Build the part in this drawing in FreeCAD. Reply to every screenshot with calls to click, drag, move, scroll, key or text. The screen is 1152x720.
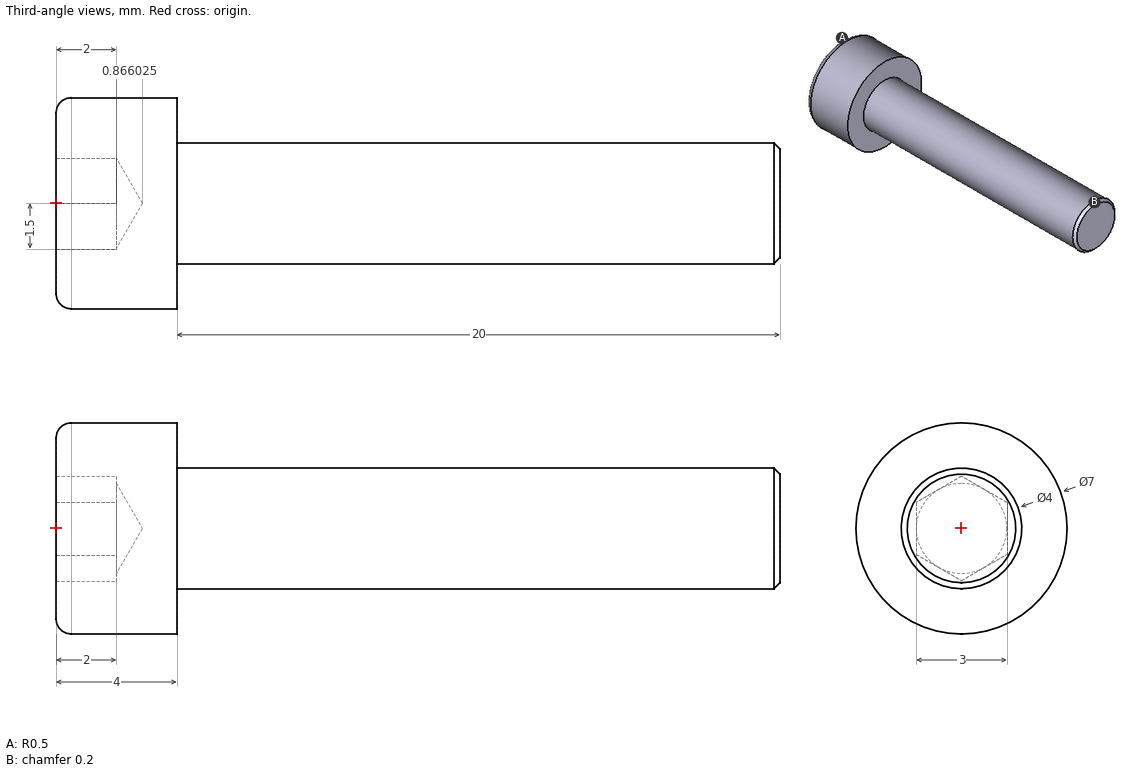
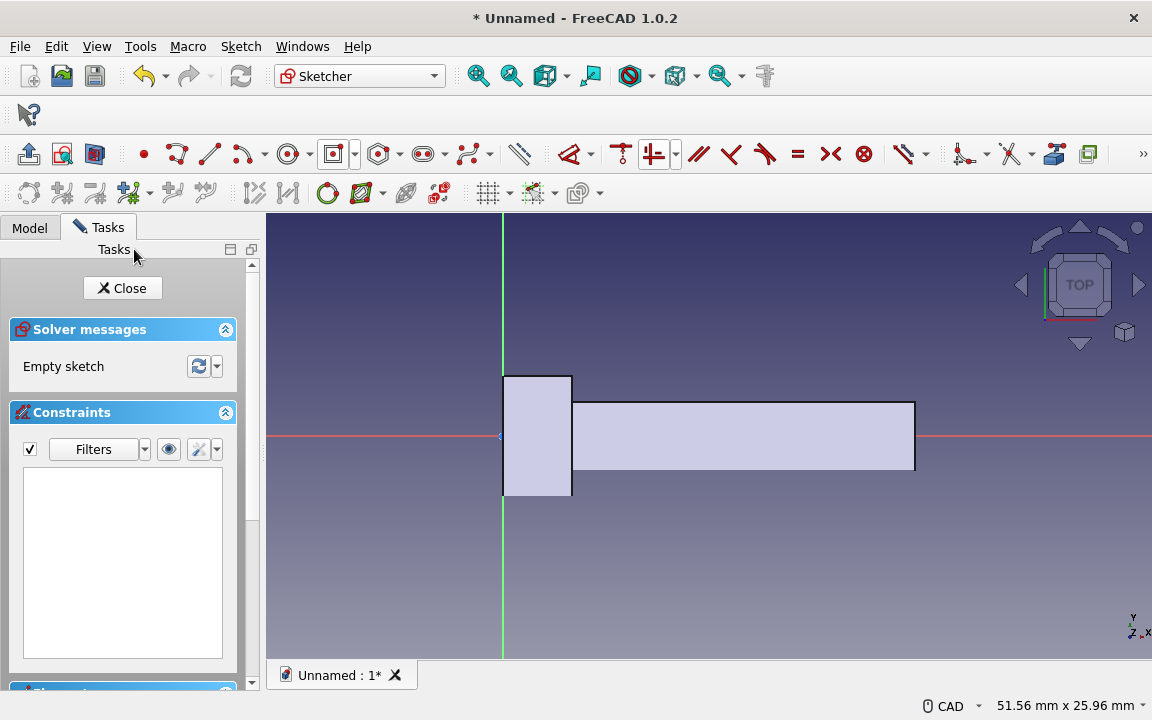
click(95, 154)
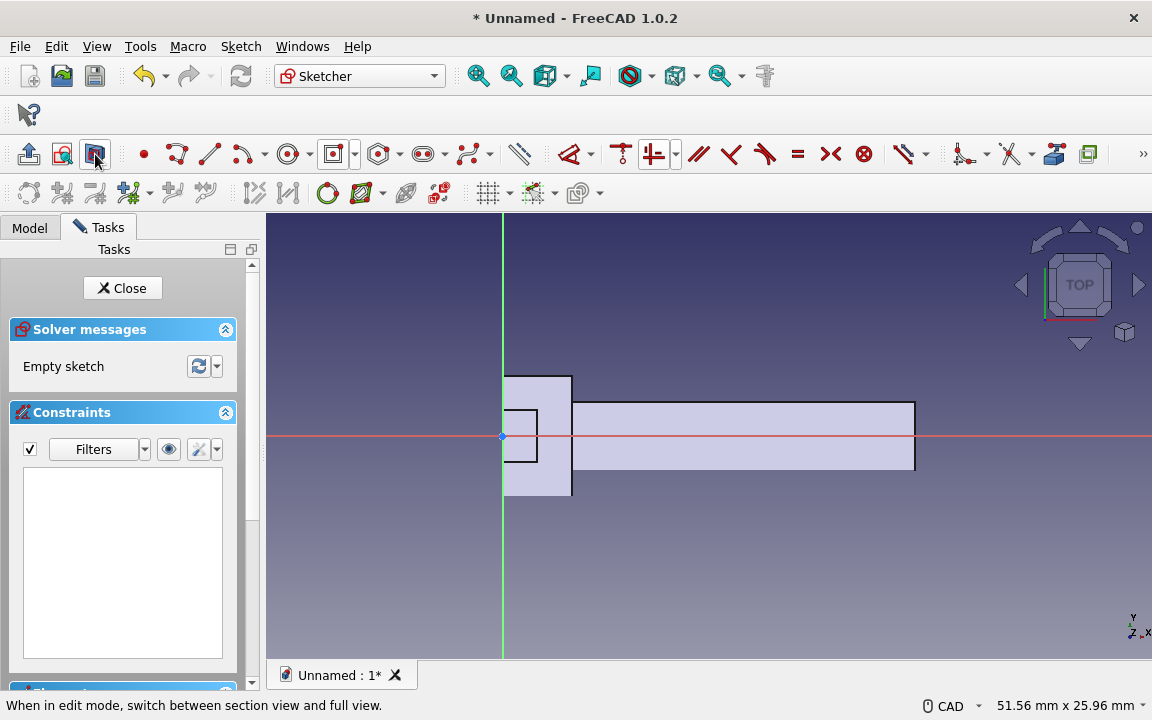
scroll(513, 451, up, 11)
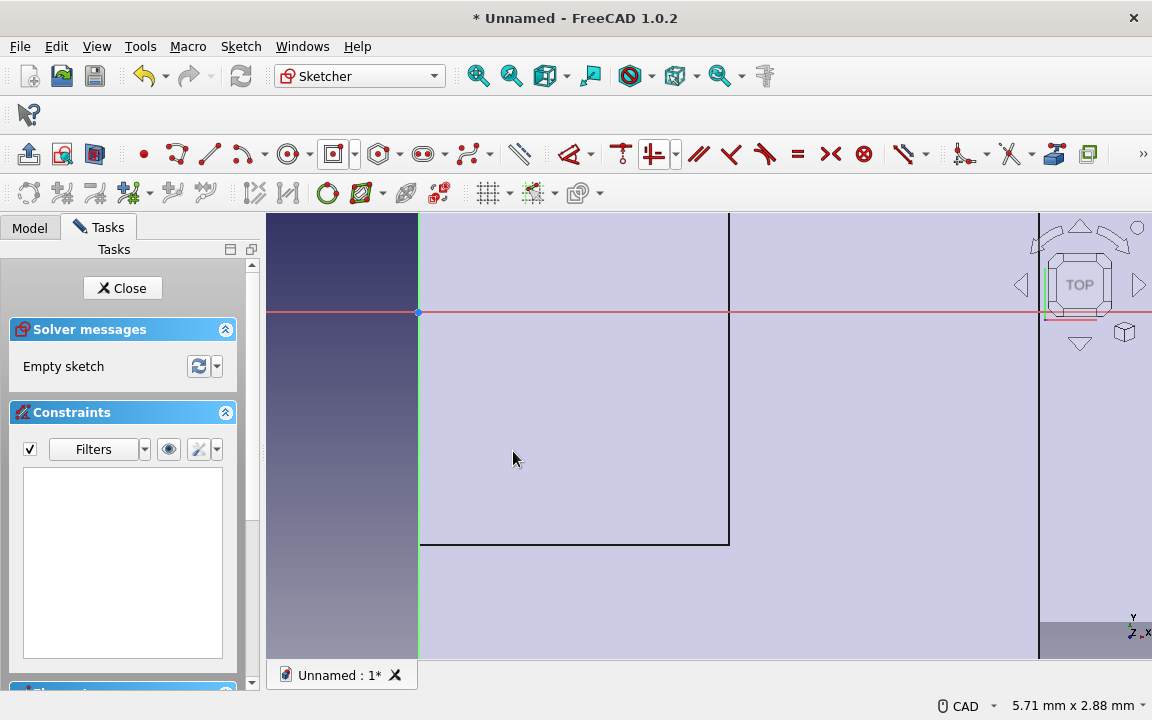
click(177, 154)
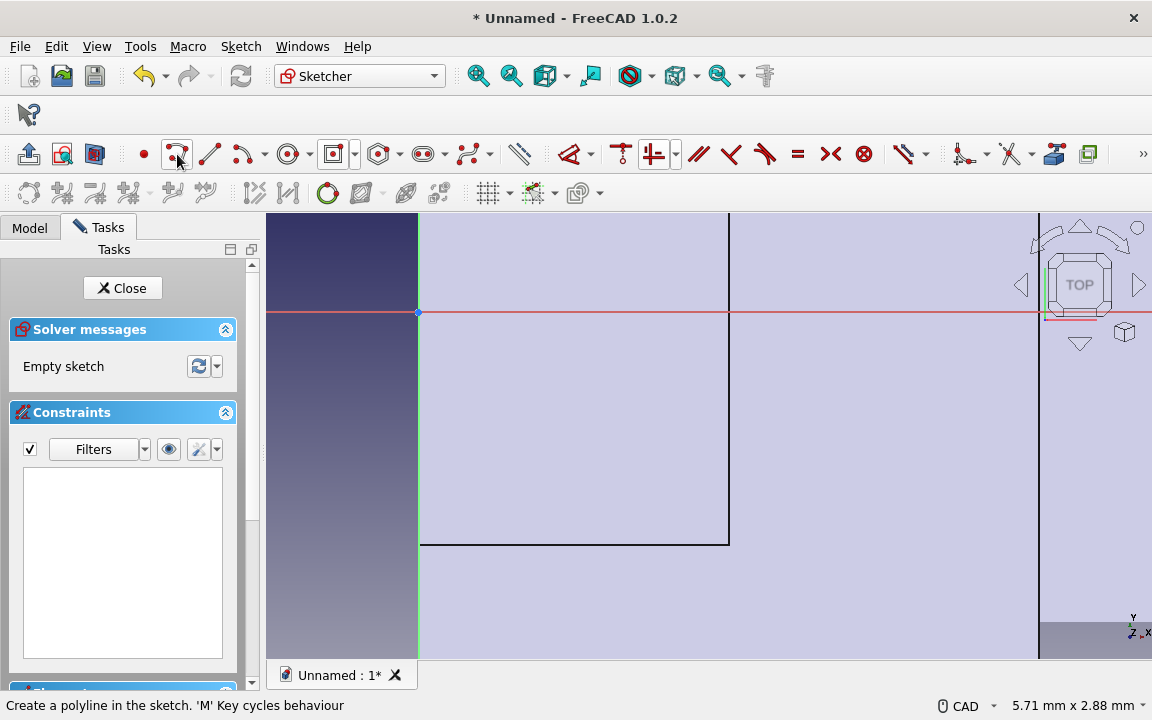
click(729, 312)
click(729, 545)
click(863, 321)
click(729, 312)
key(Escape)
key(Escape)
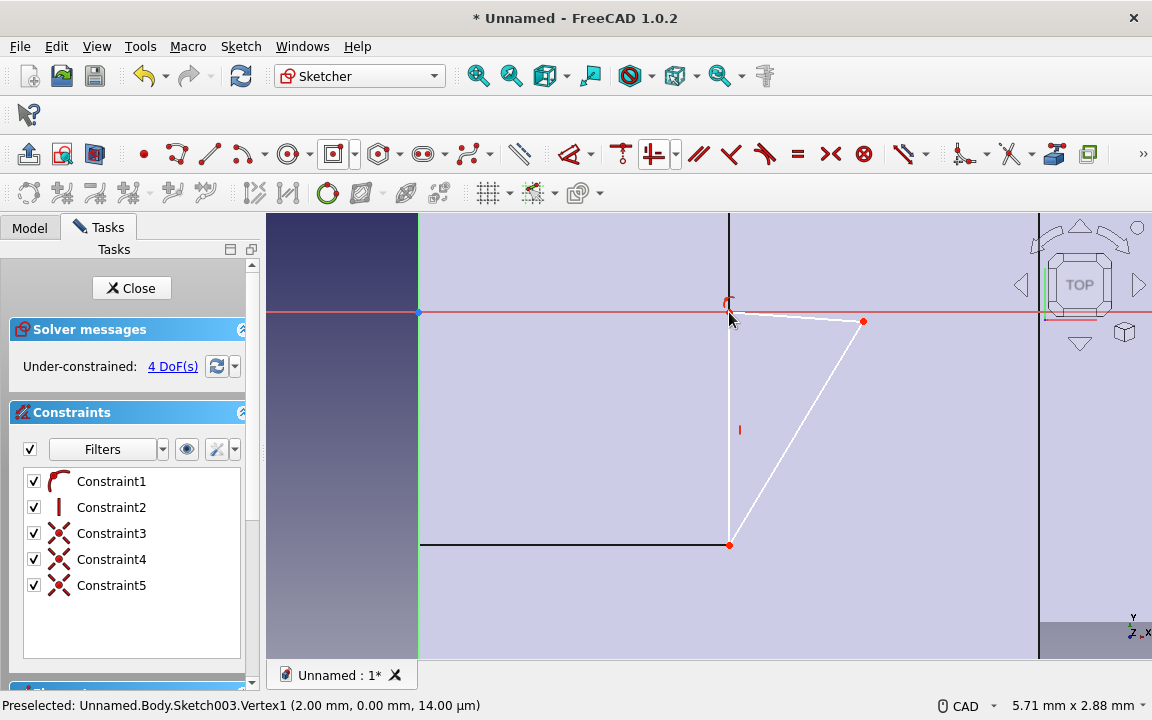
click(769, 315)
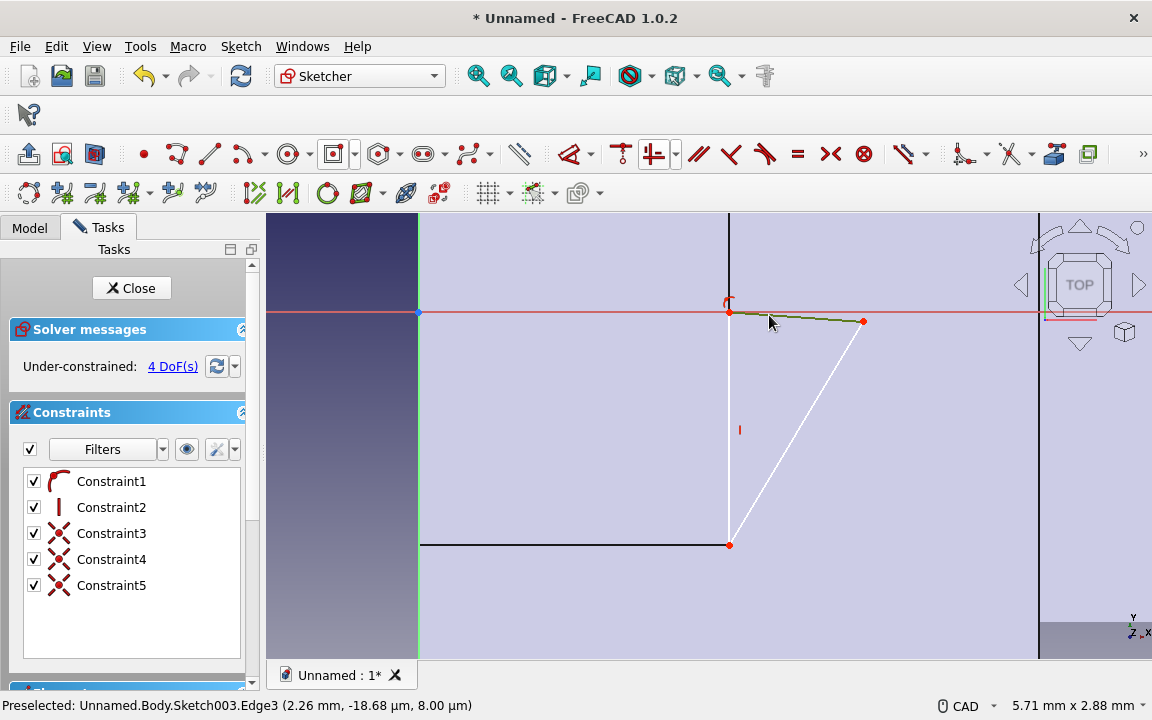
click(676, 154)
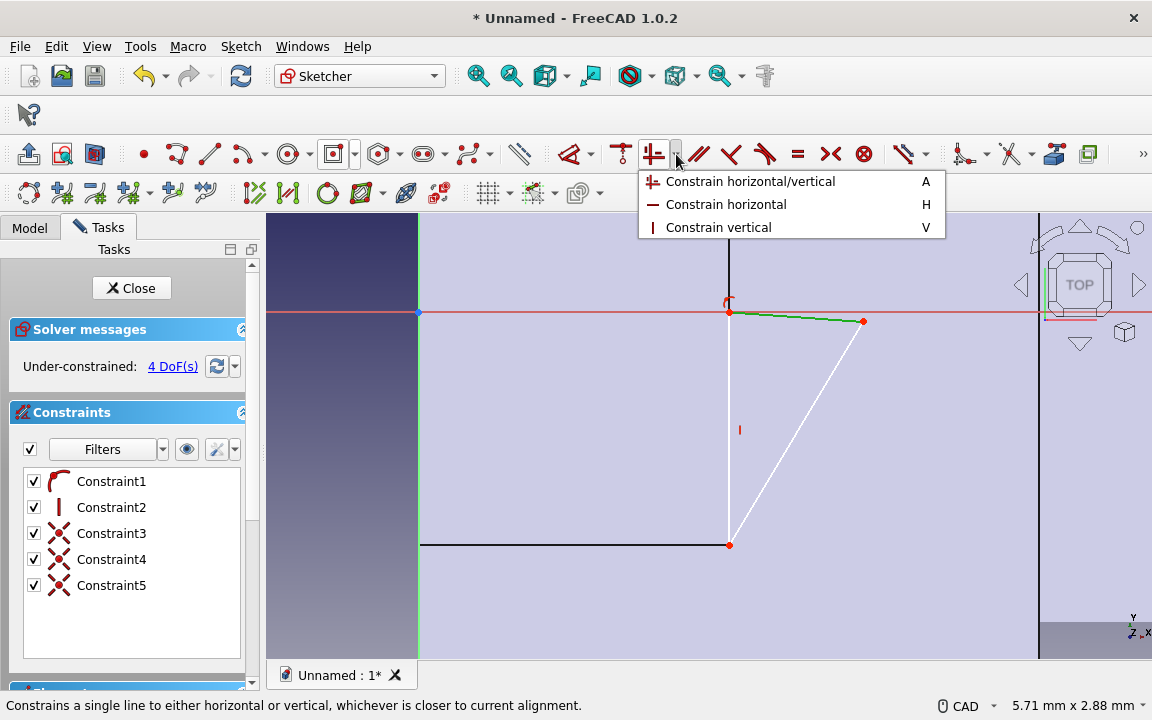
click(792, 204)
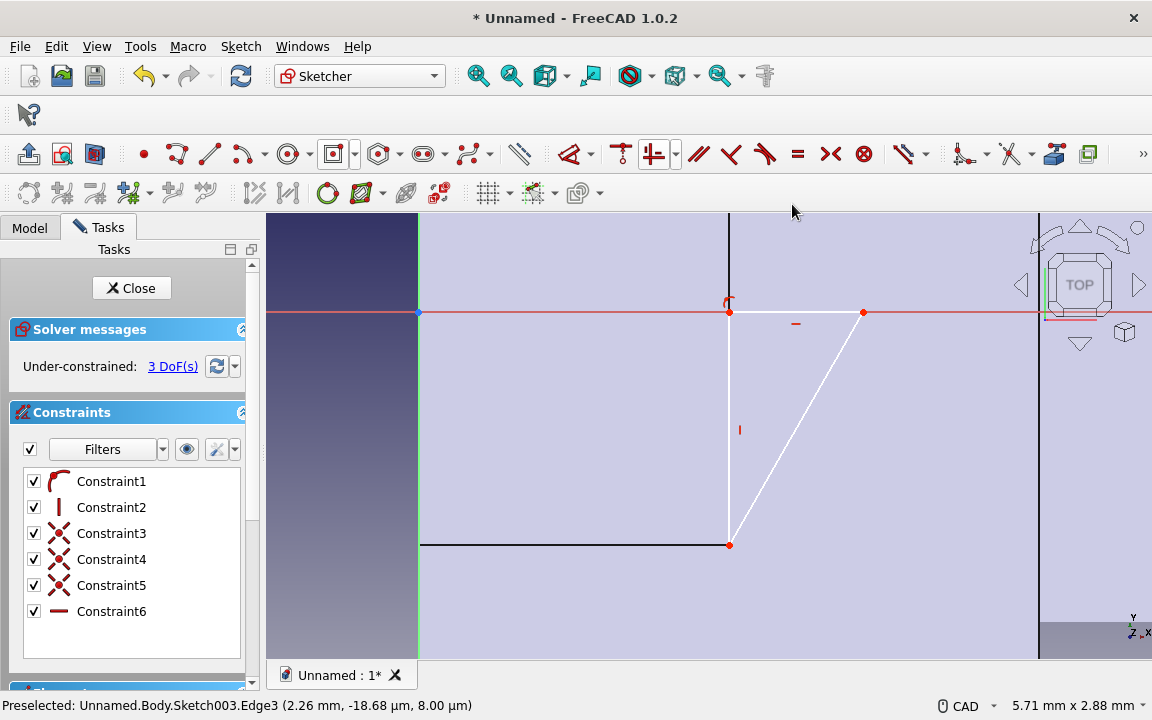
click(568, 154)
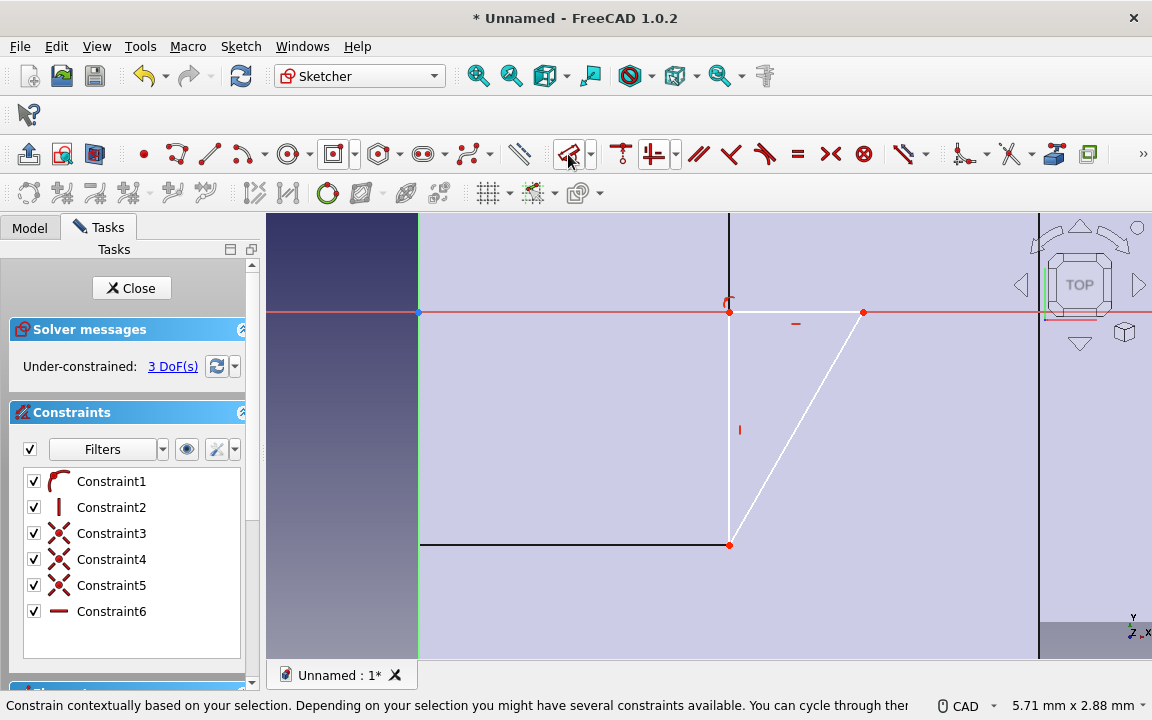
click(729, 312)
click(574, 278)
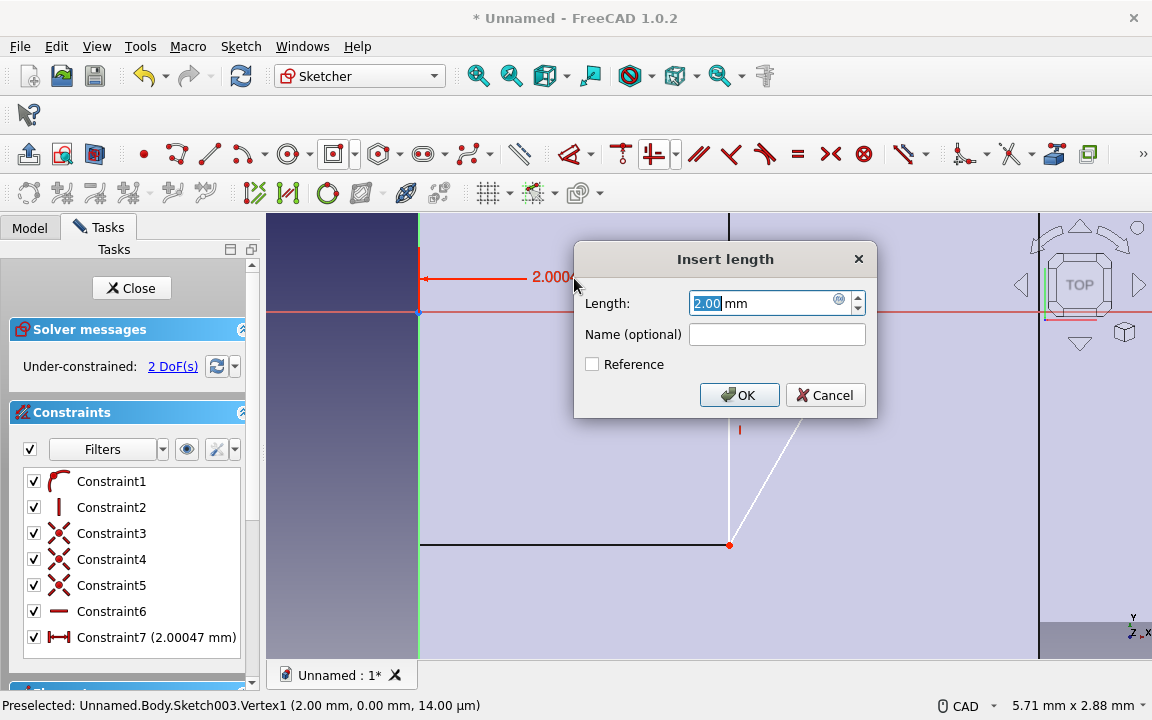
text(2)
key(Return)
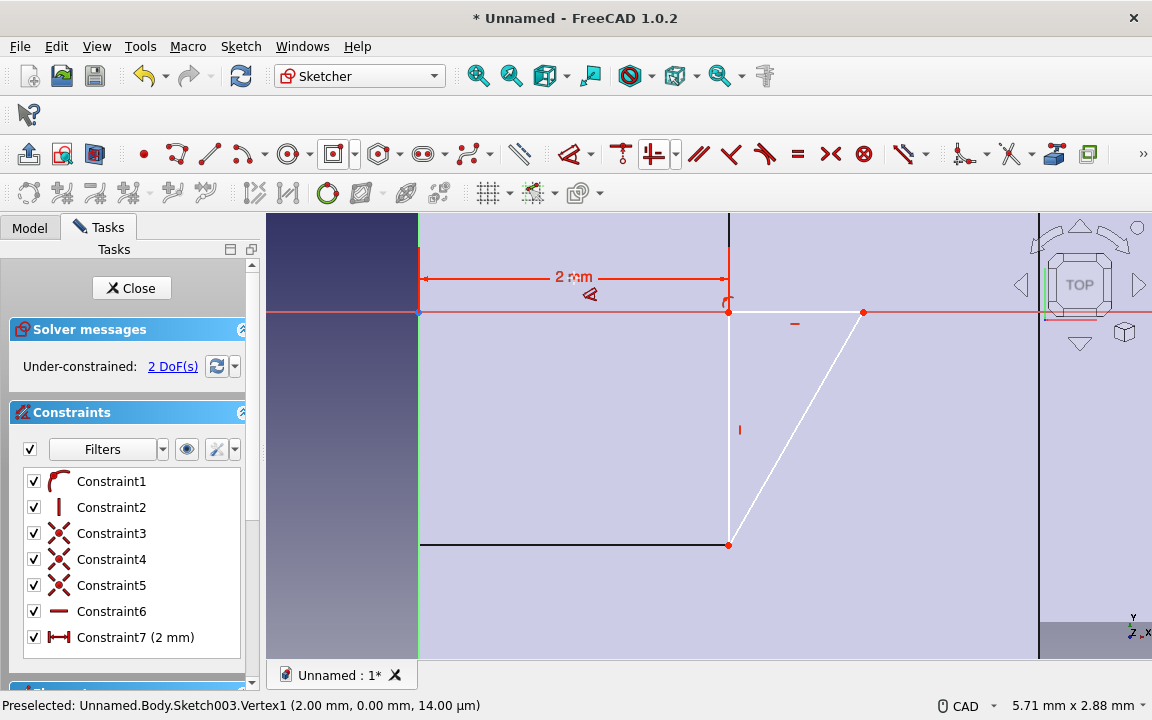
click(729, 382)
click(763, 429)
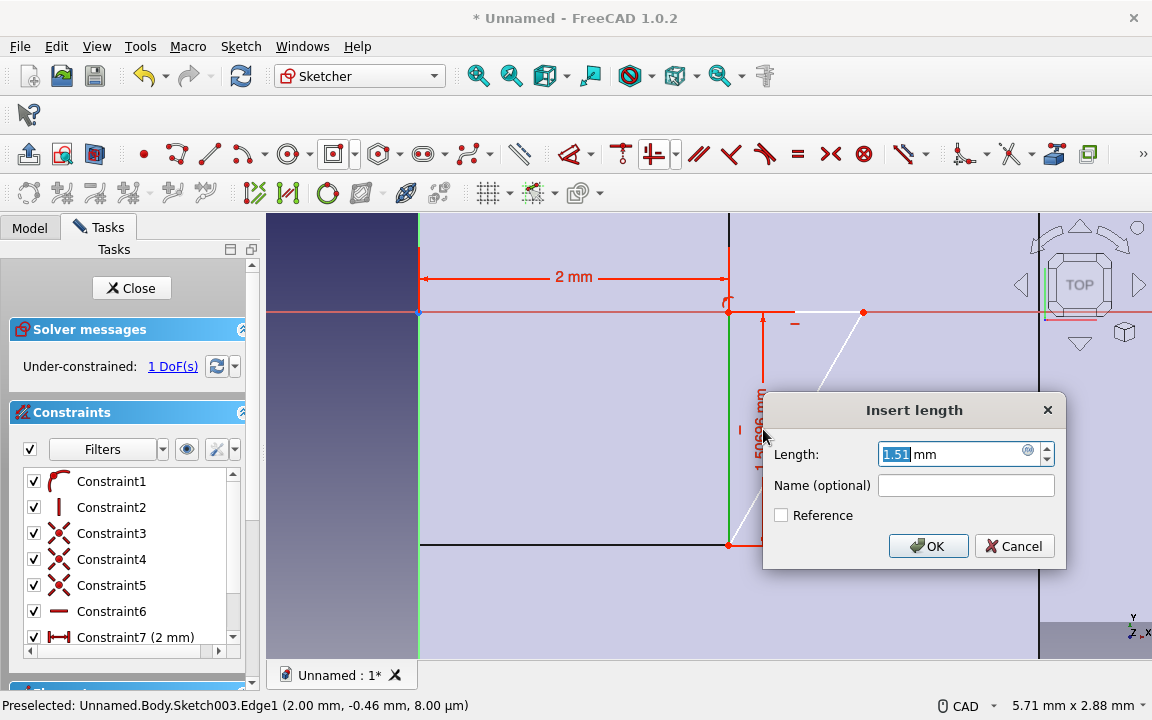
text(1.5)
key(Return)